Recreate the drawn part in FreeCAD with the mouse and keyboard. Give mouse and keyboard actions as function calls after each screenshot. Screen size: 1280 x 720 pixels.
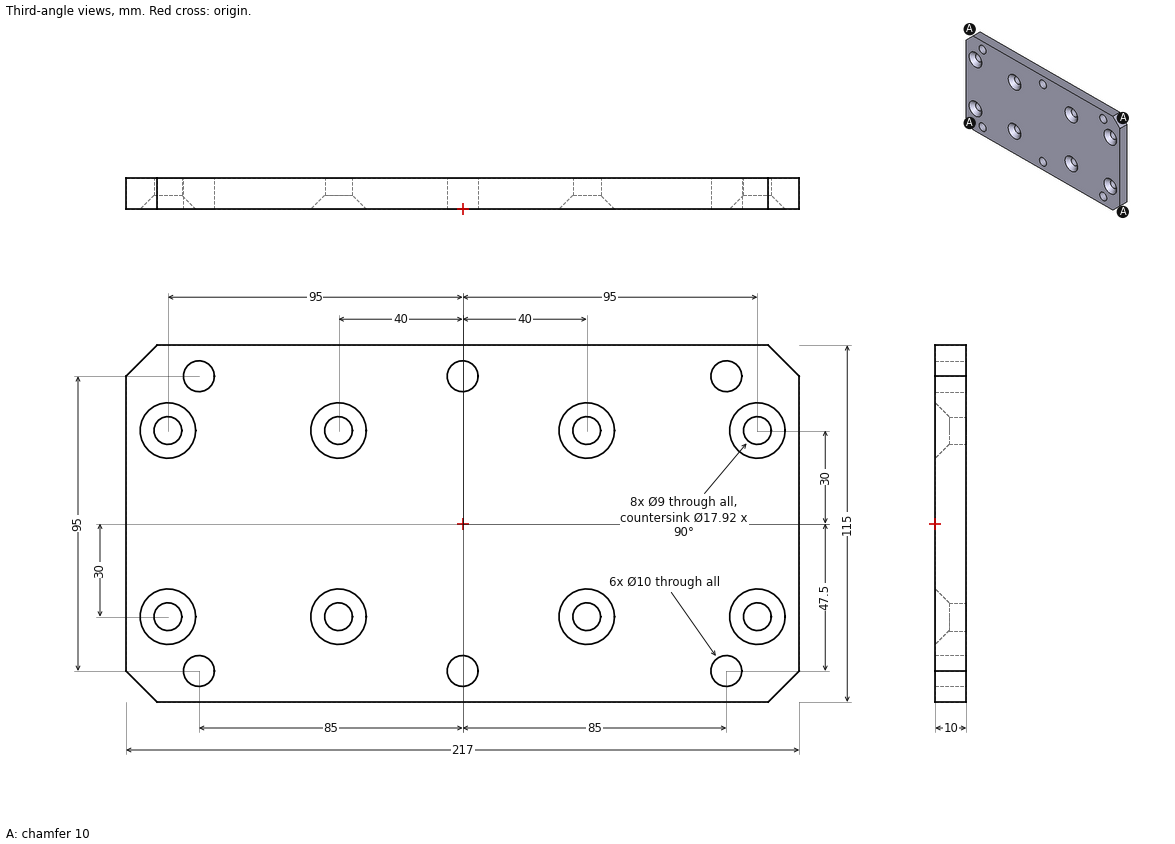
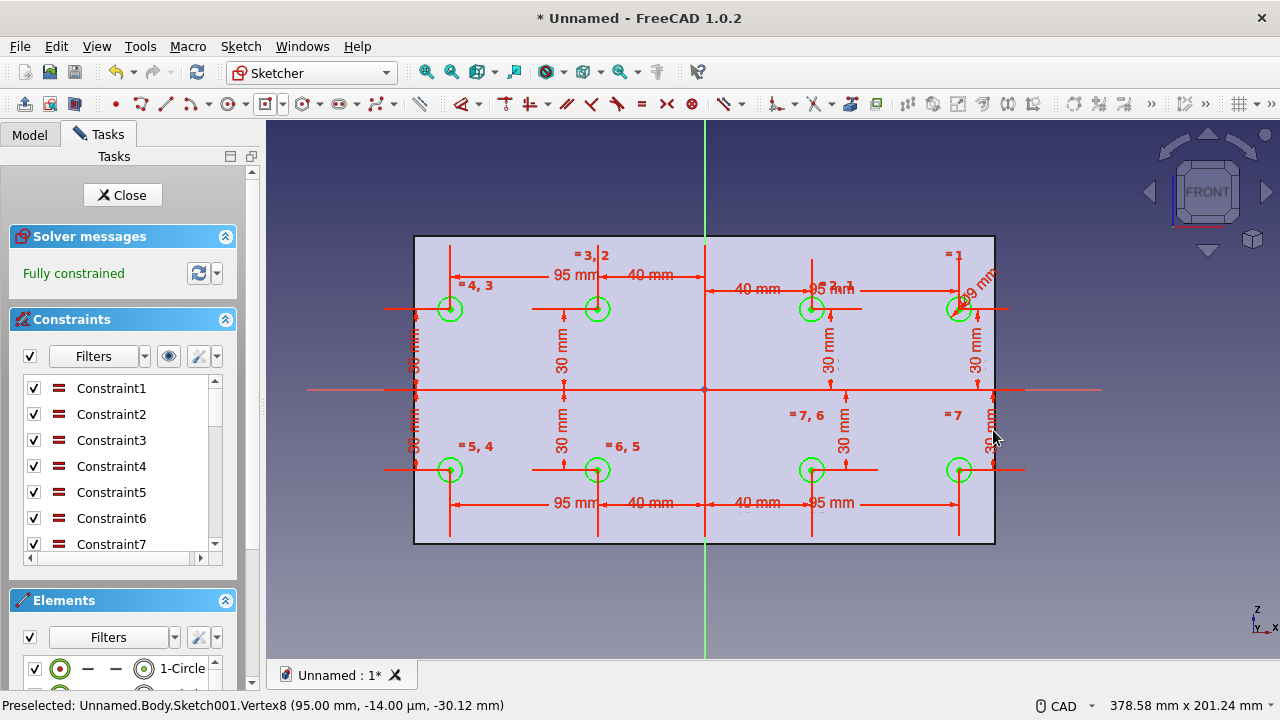
click(123, 195)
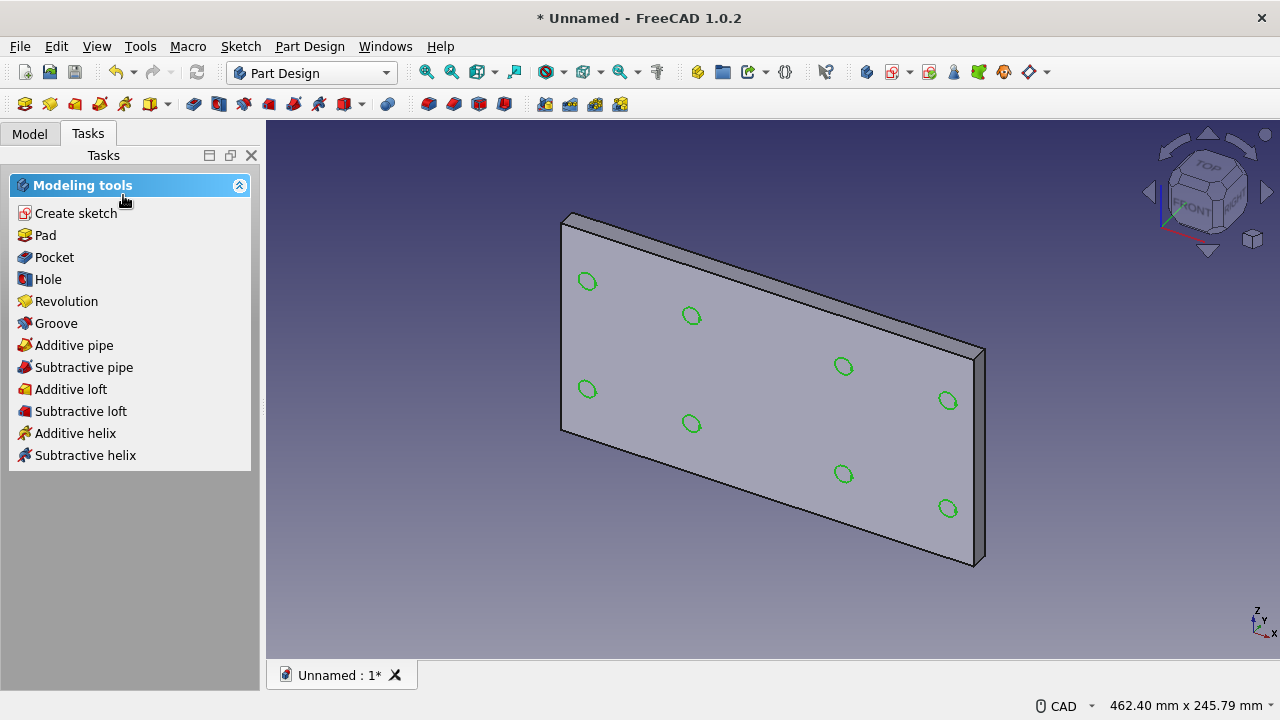
click(219, 104)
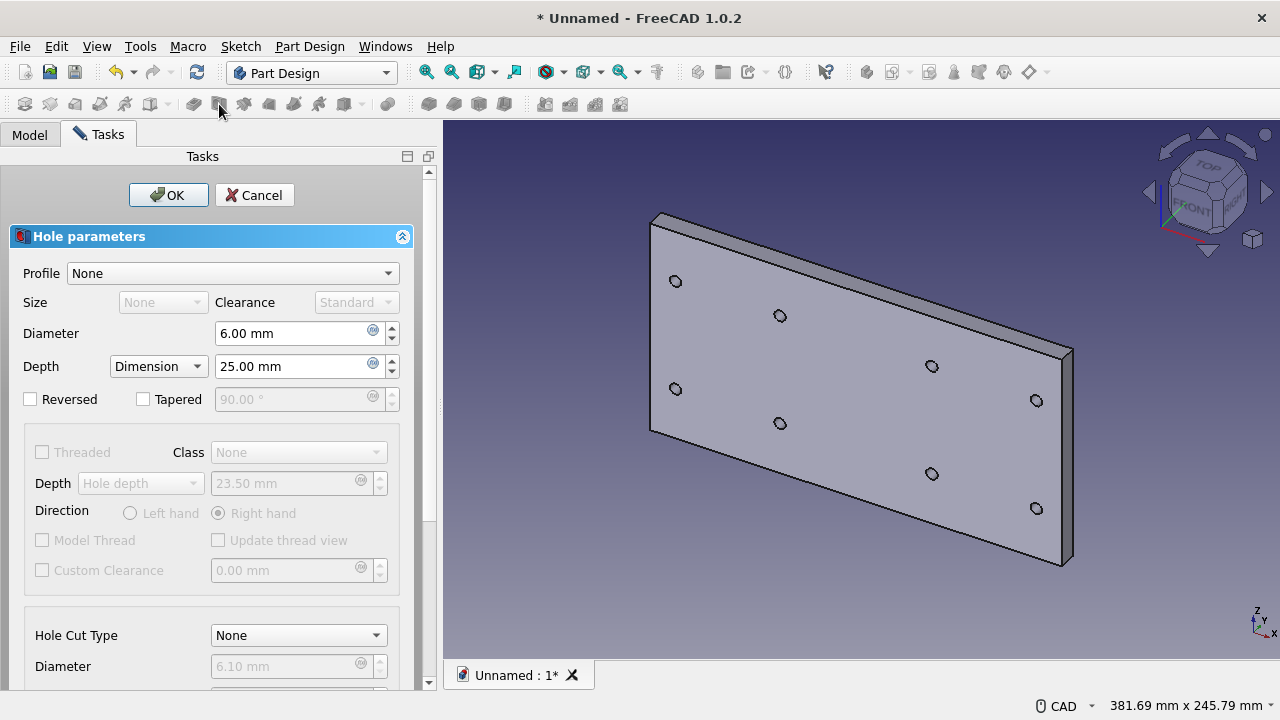
triple_click(300, 334)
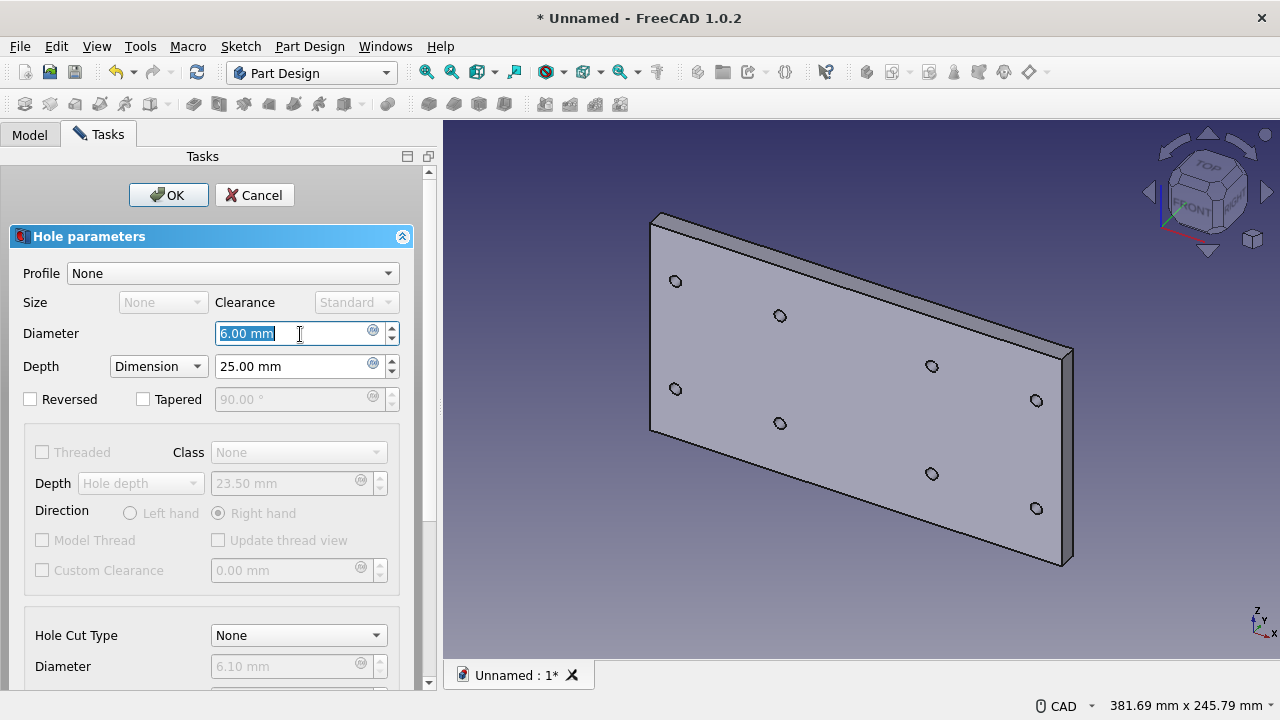
text(9)
key(Tab)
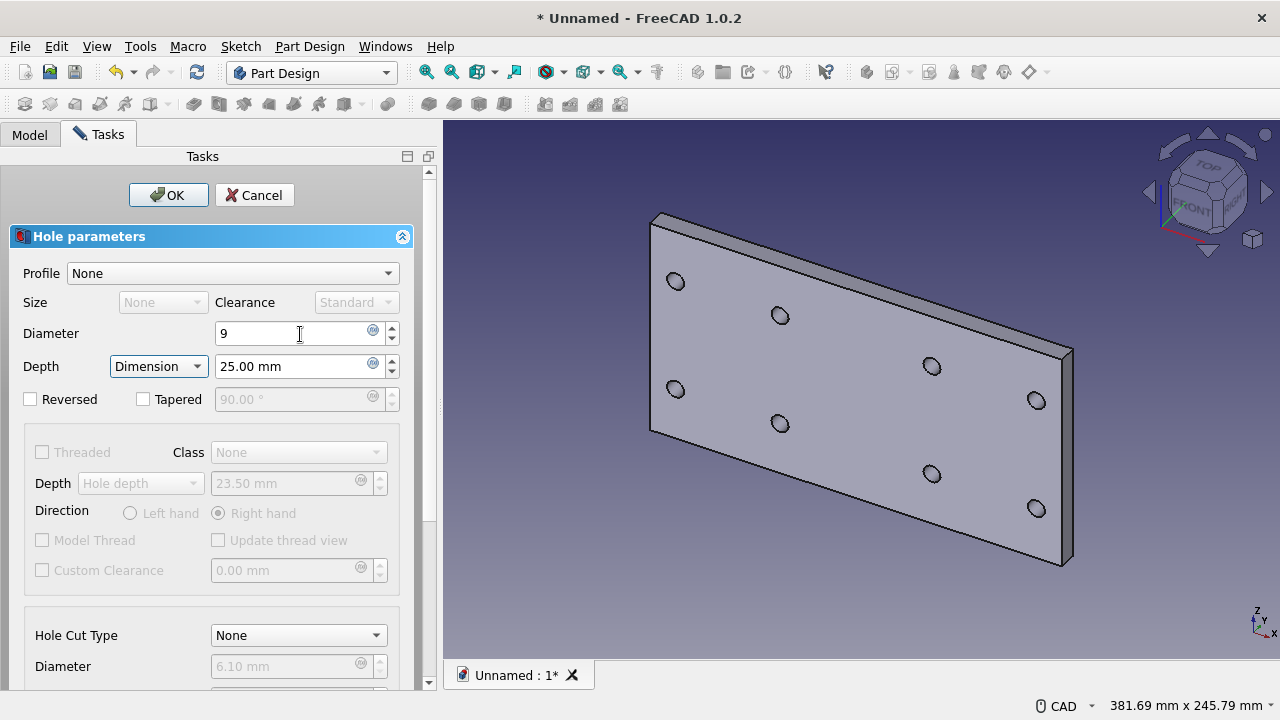
click(160, 366)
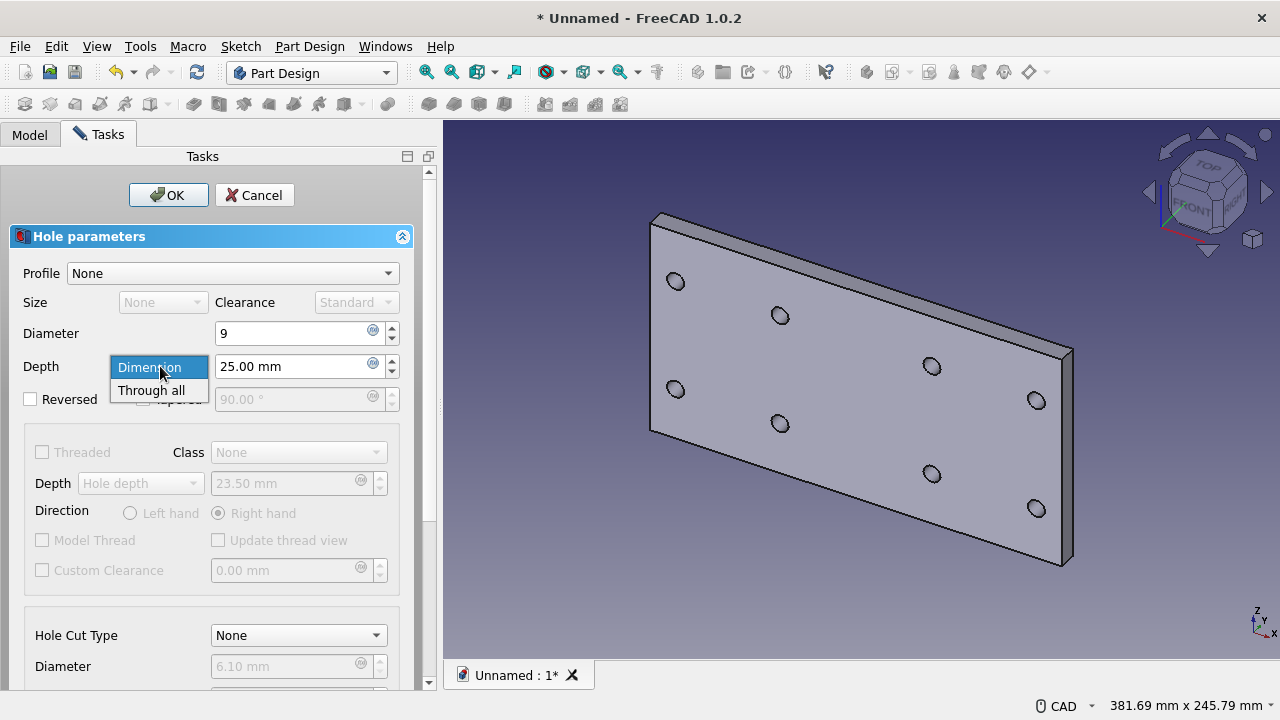
click(158, 390)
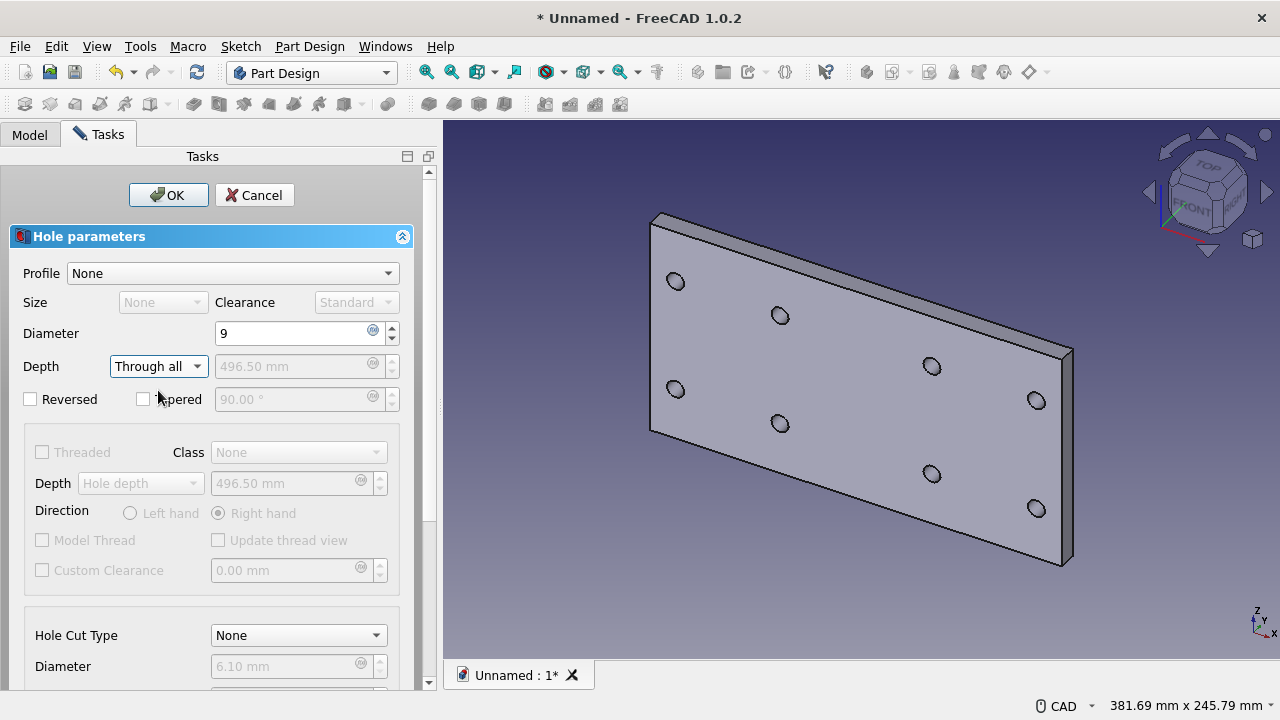
click(300, 636)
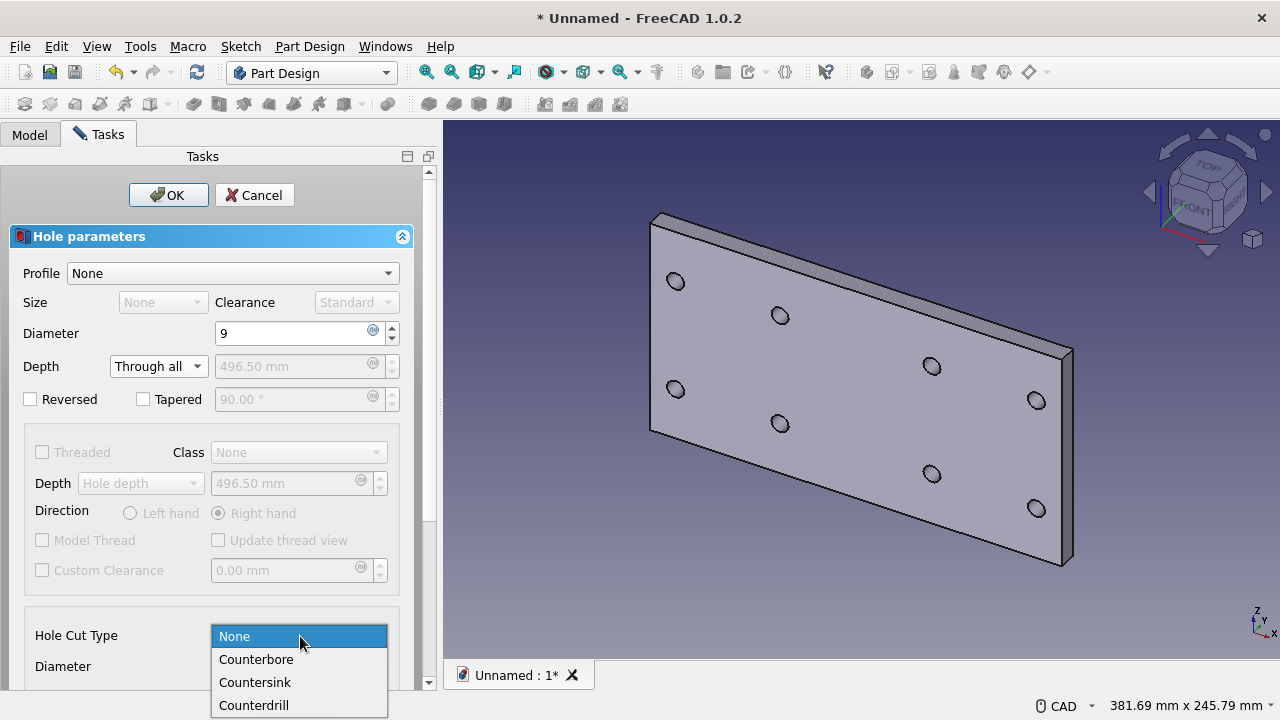
click(298, 682)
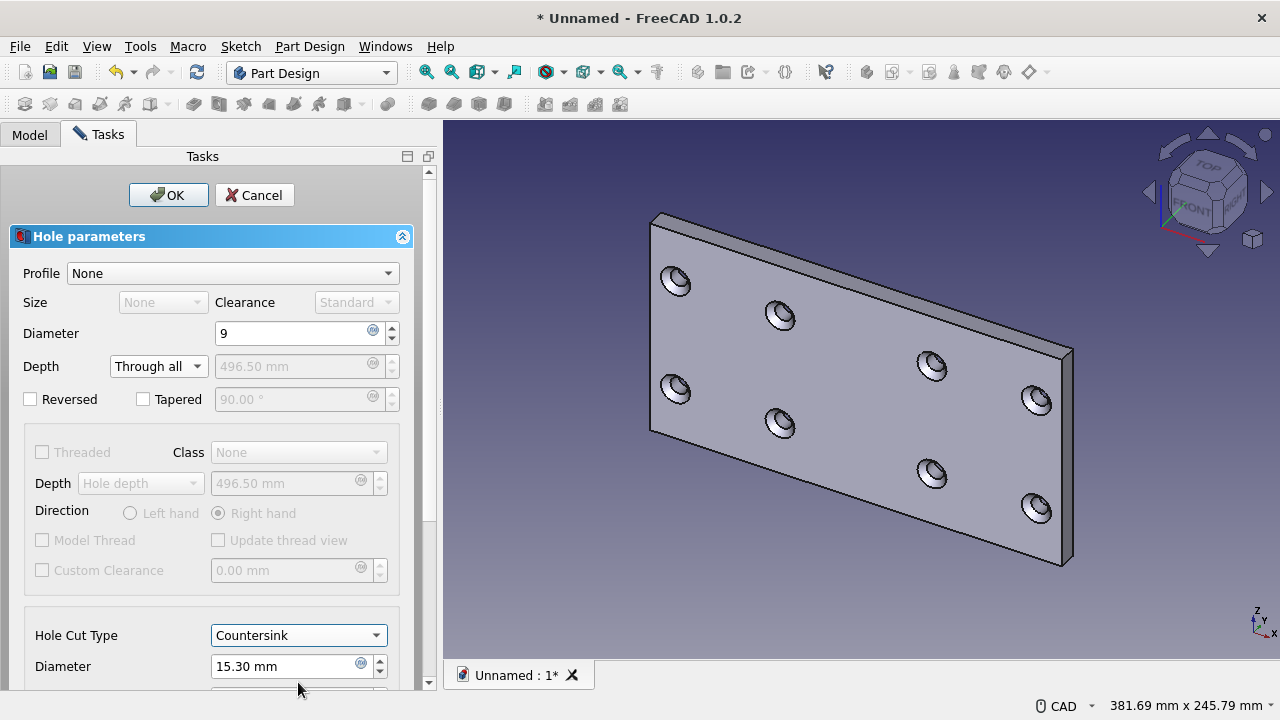
triple_click(292, 666)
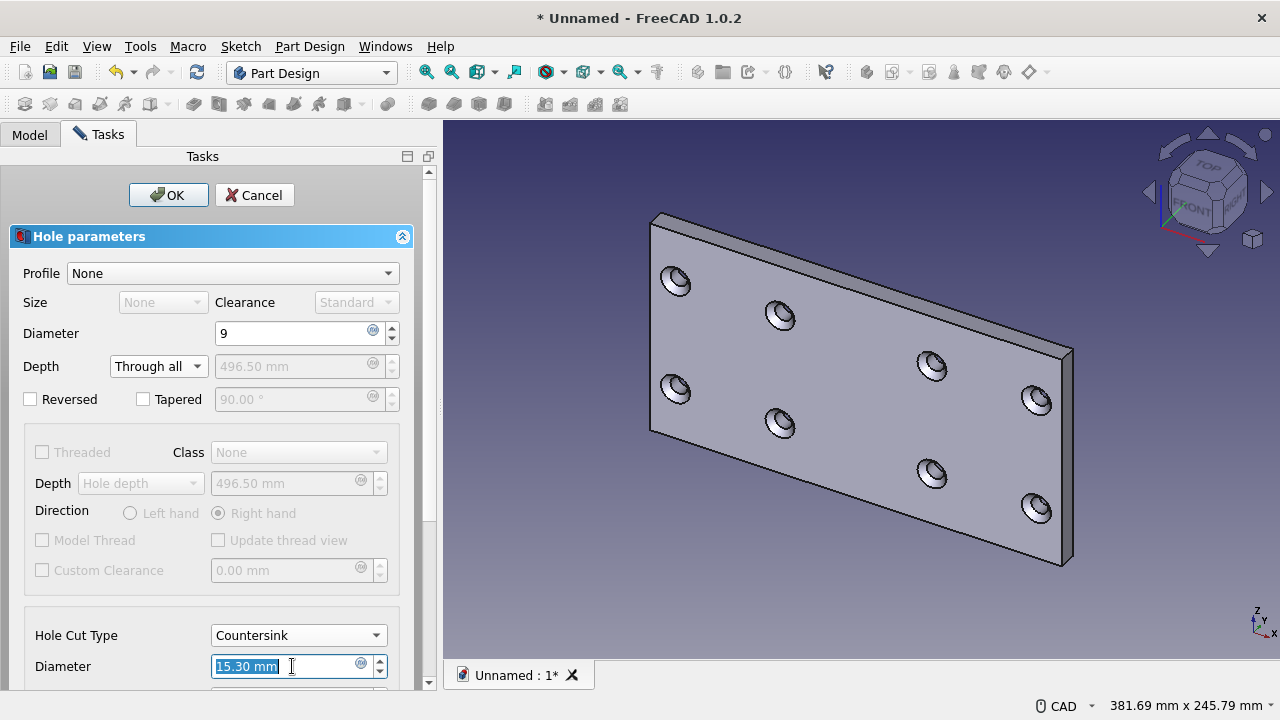
text(17.92)
key(Tab)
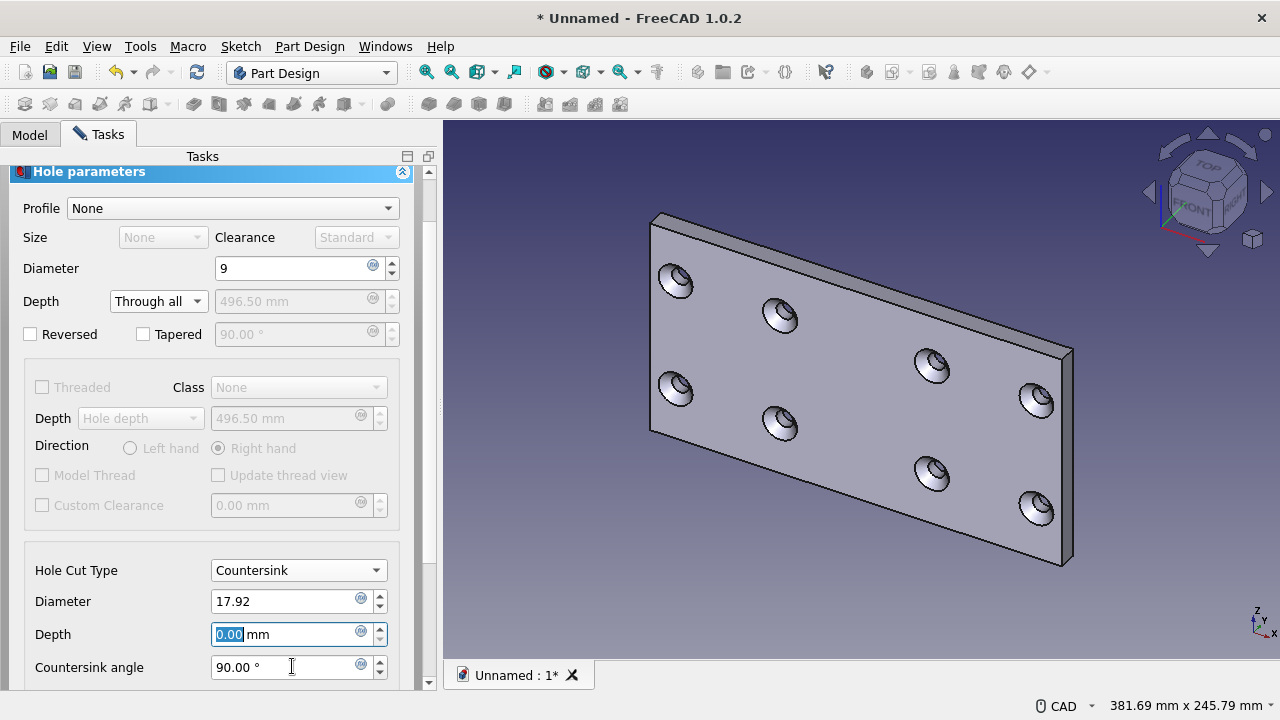
scroll(429, 428, up, 2)